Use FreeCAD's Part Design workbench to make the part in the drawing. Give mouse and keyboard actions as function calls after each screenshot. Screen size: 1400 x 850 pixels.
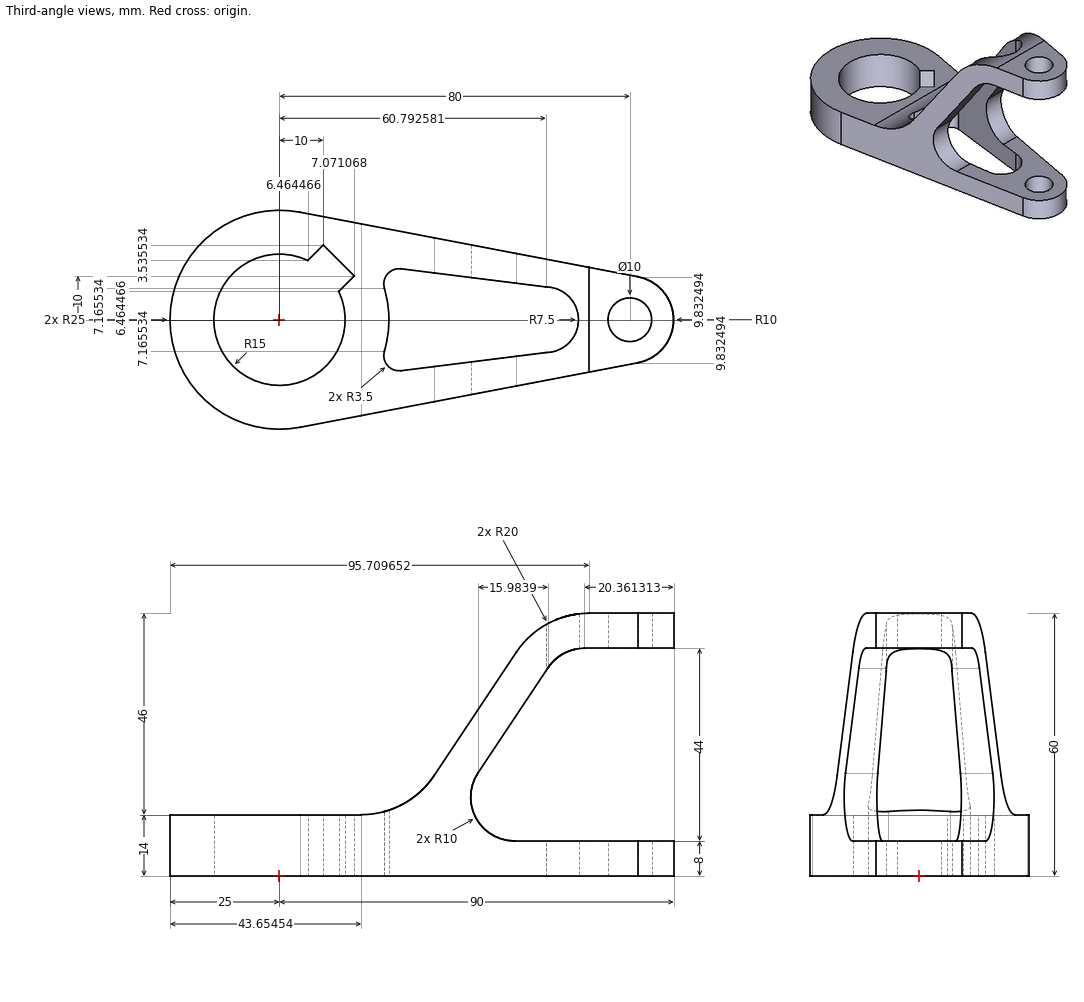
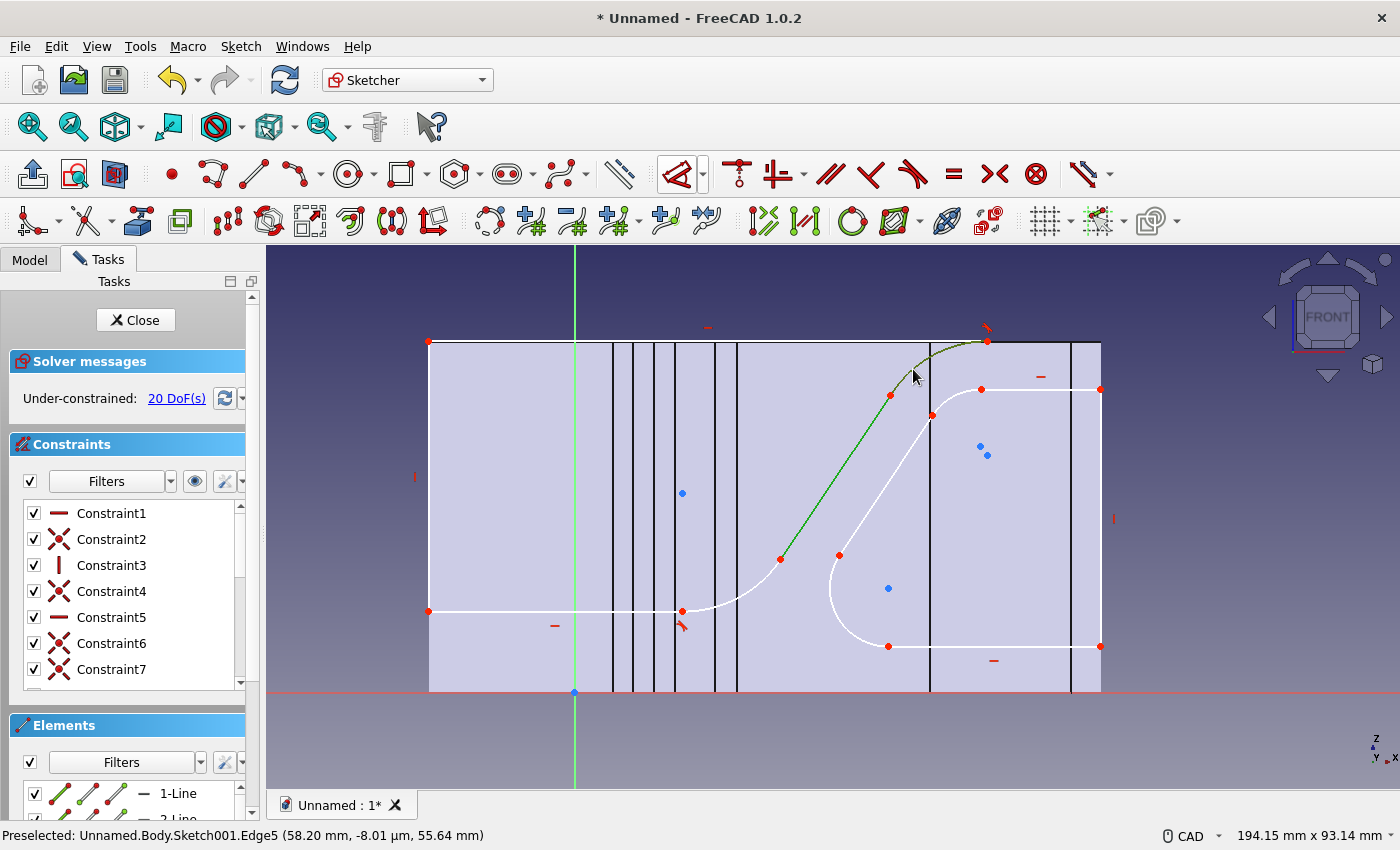
key(t)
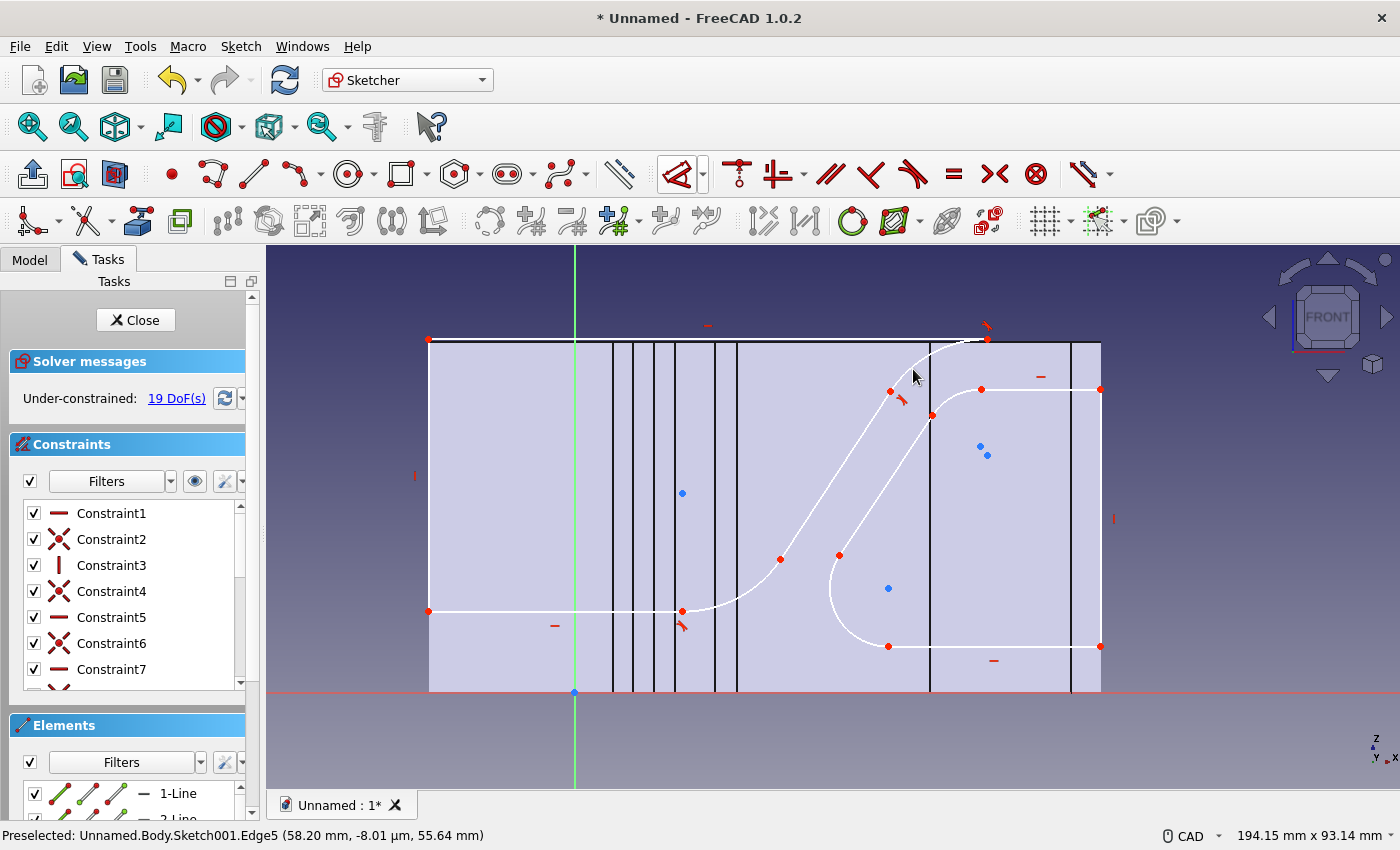
click(858, 442)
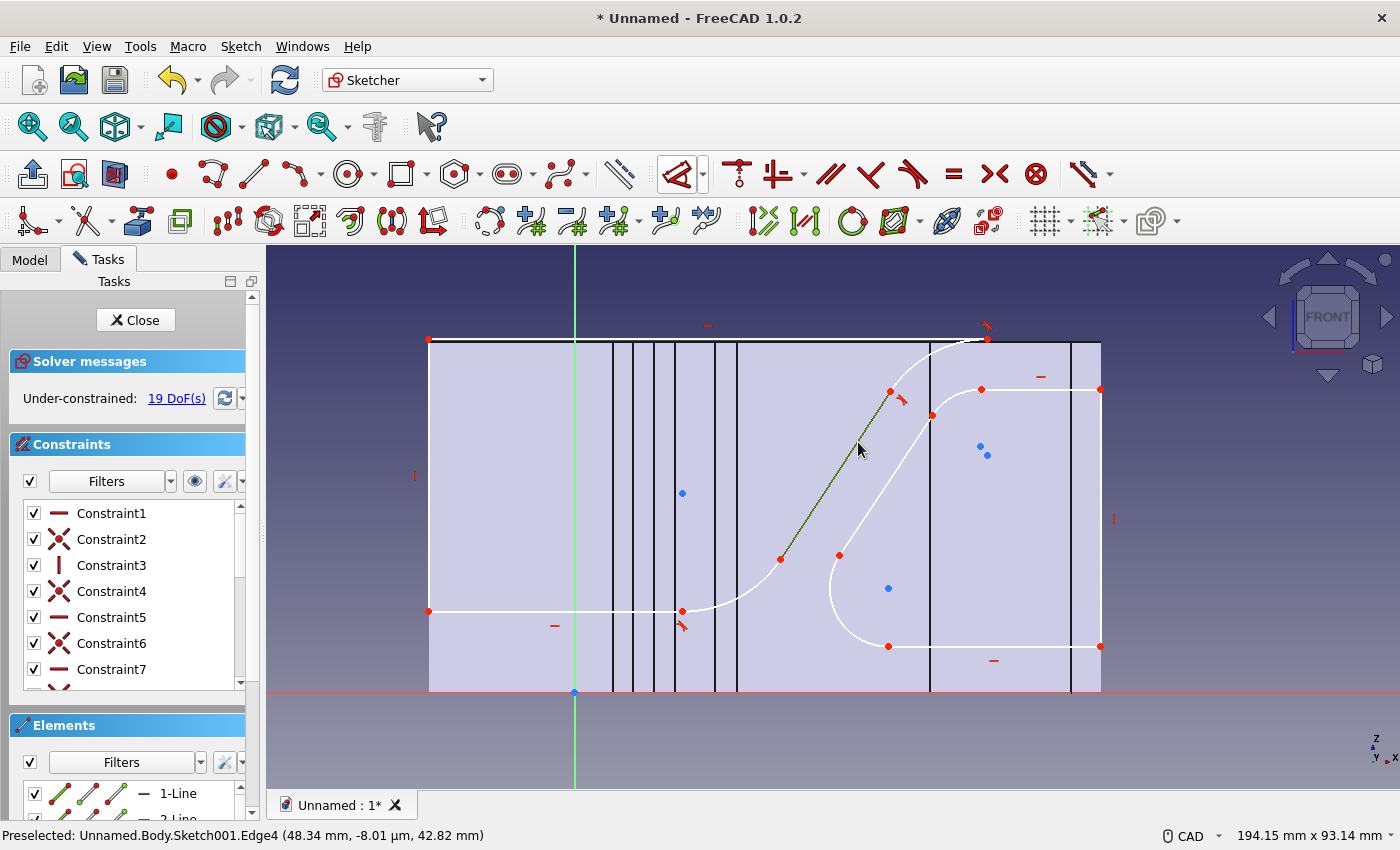
click(717, 607)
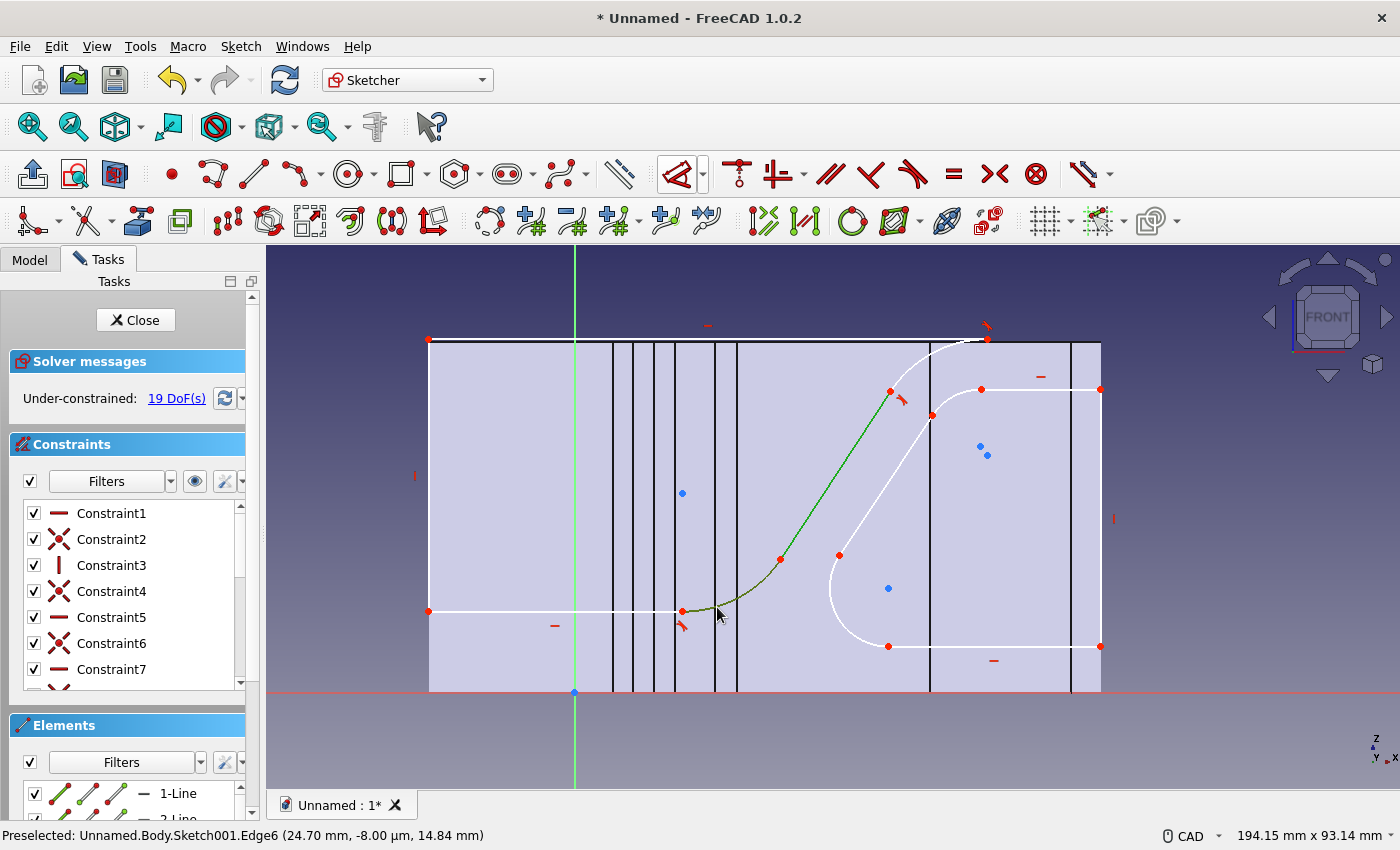
click(913, 174)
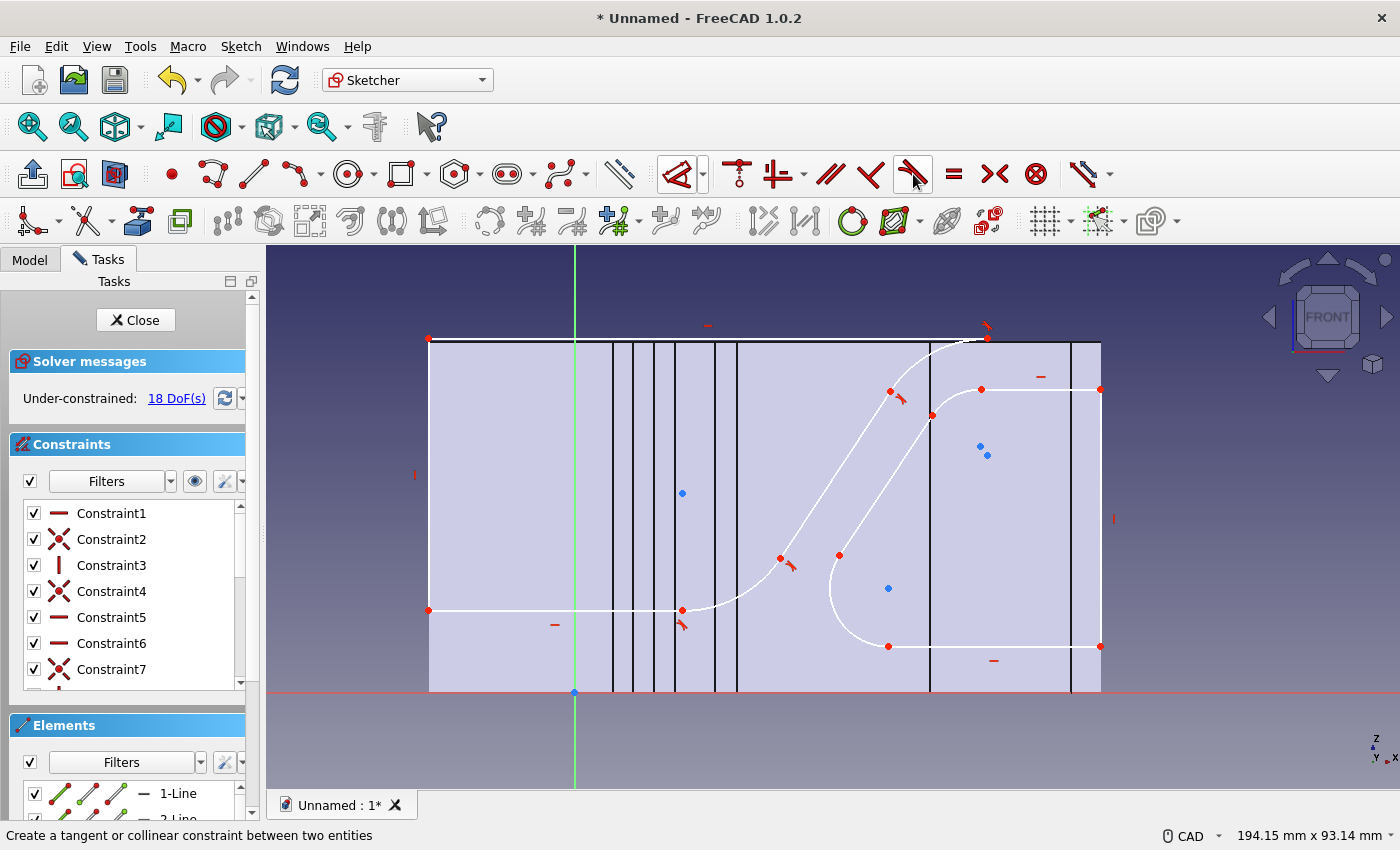
click(868, 514)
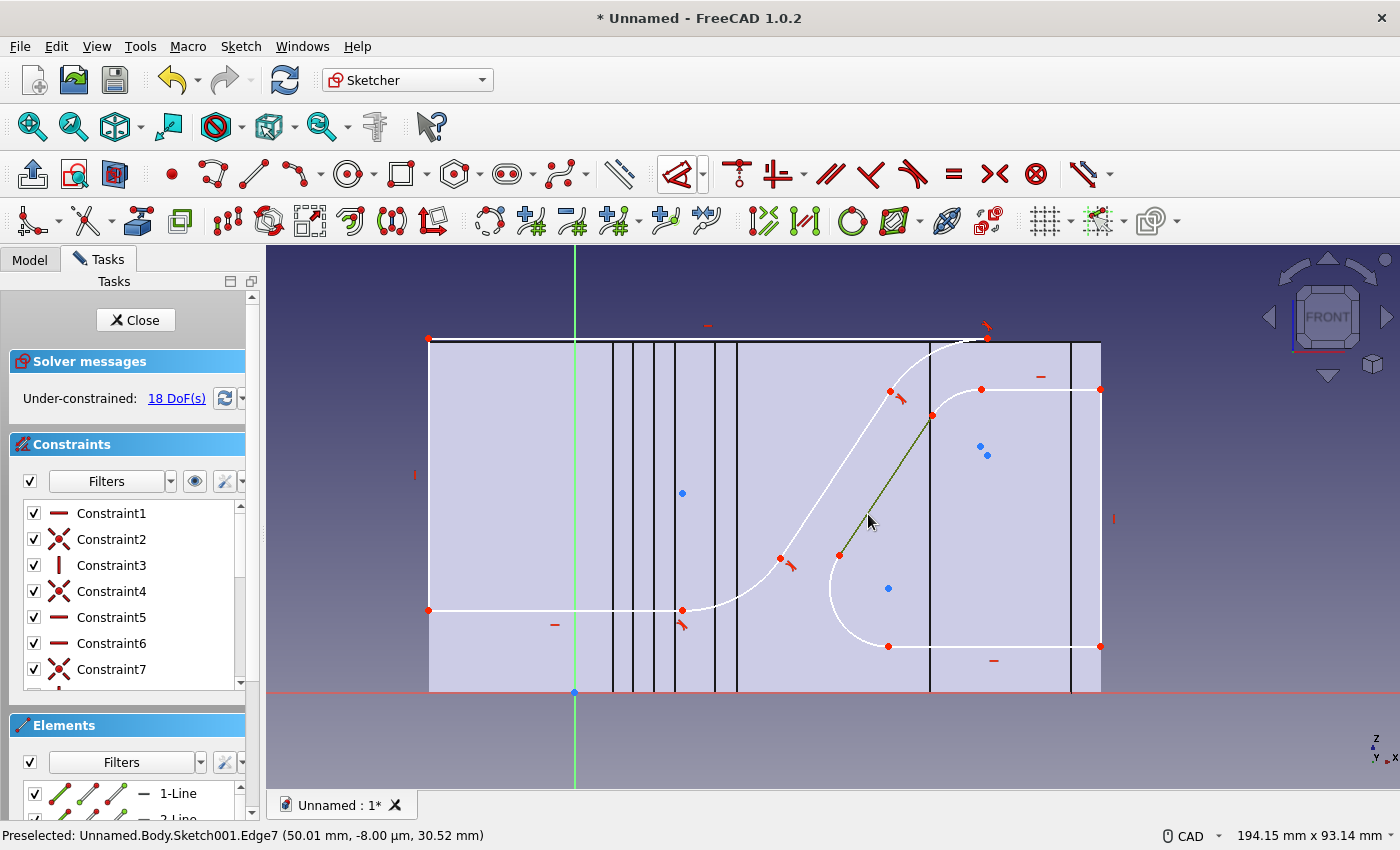
click(964, 392)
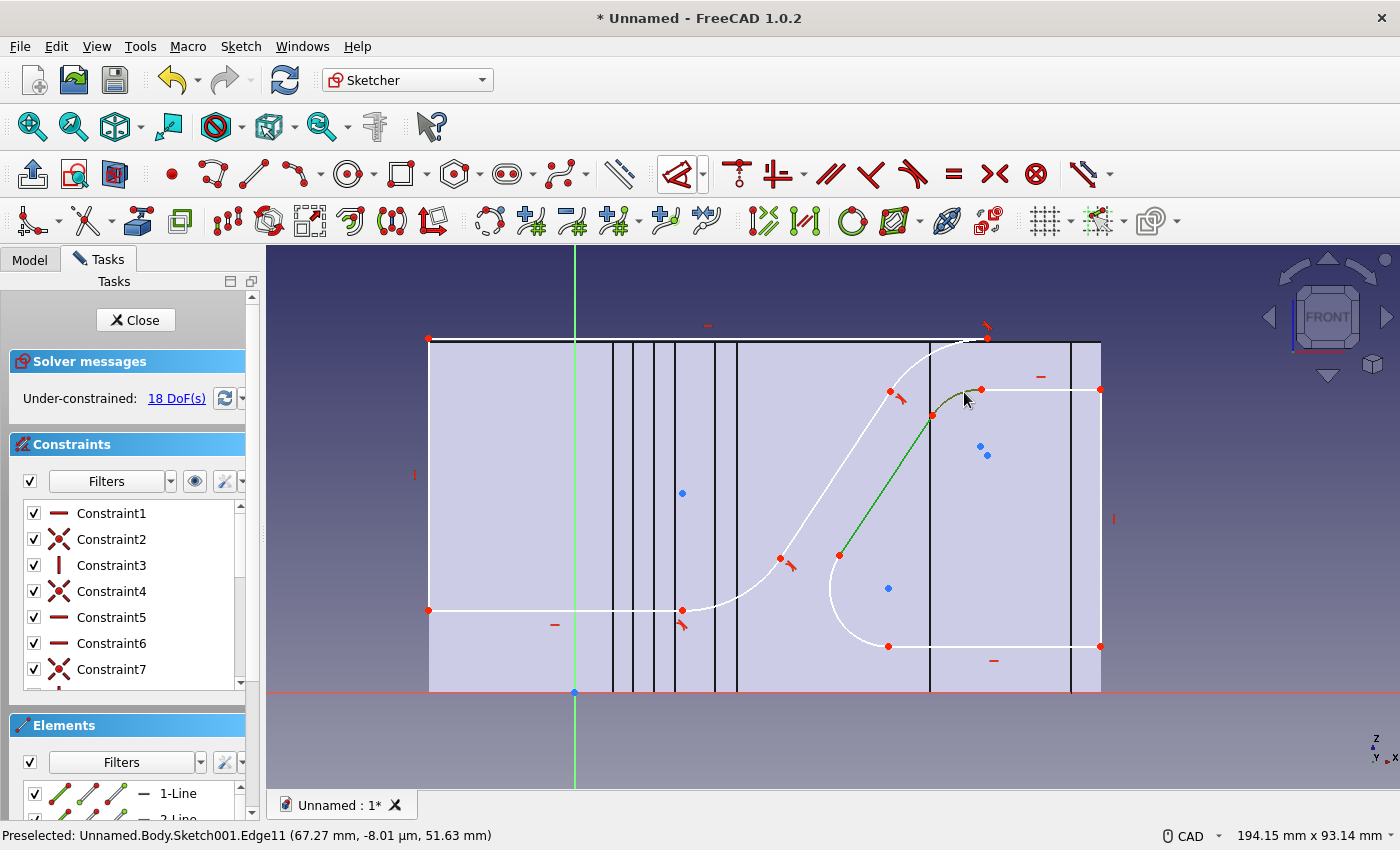
click(913, 174)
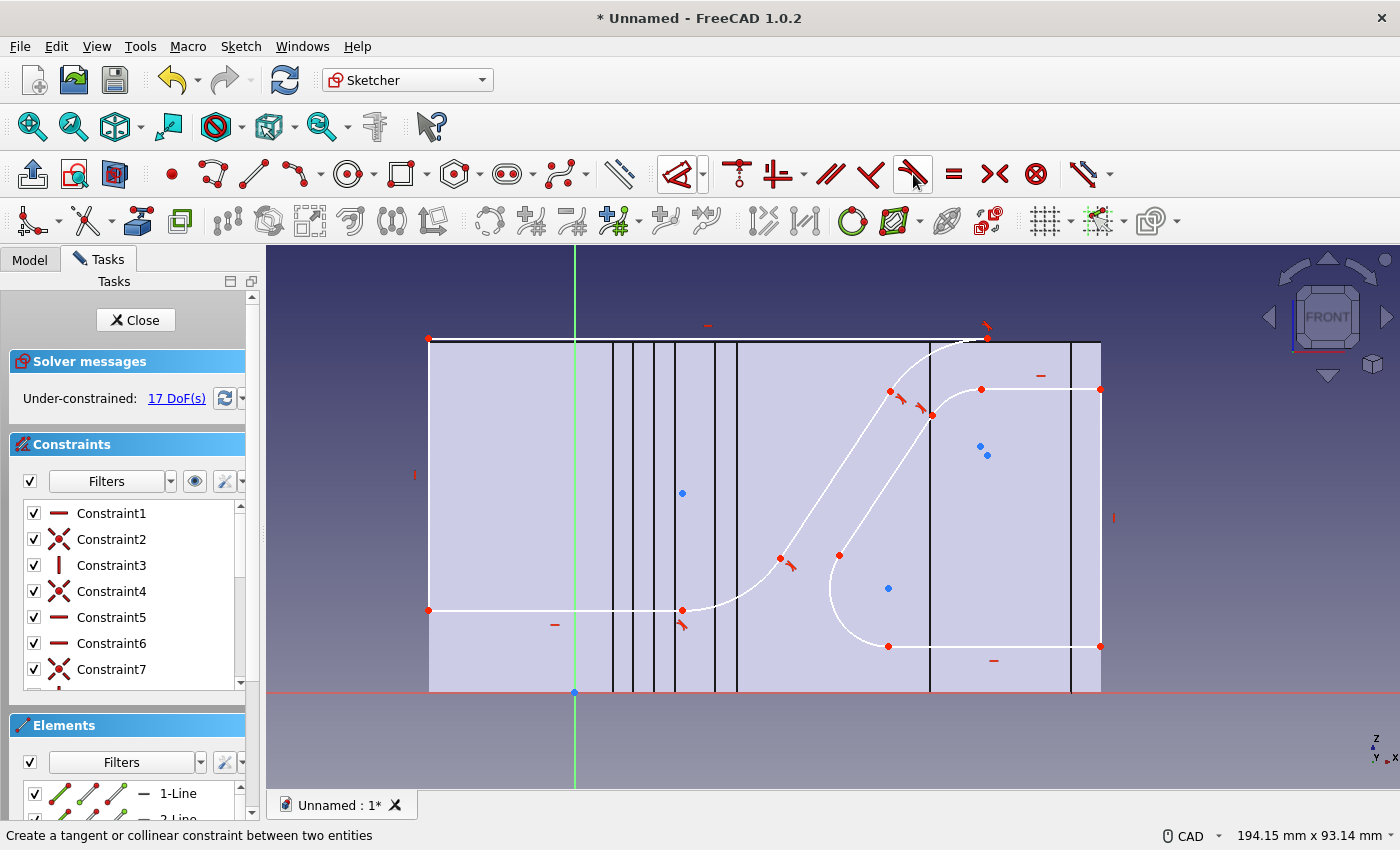
click(868, 513)